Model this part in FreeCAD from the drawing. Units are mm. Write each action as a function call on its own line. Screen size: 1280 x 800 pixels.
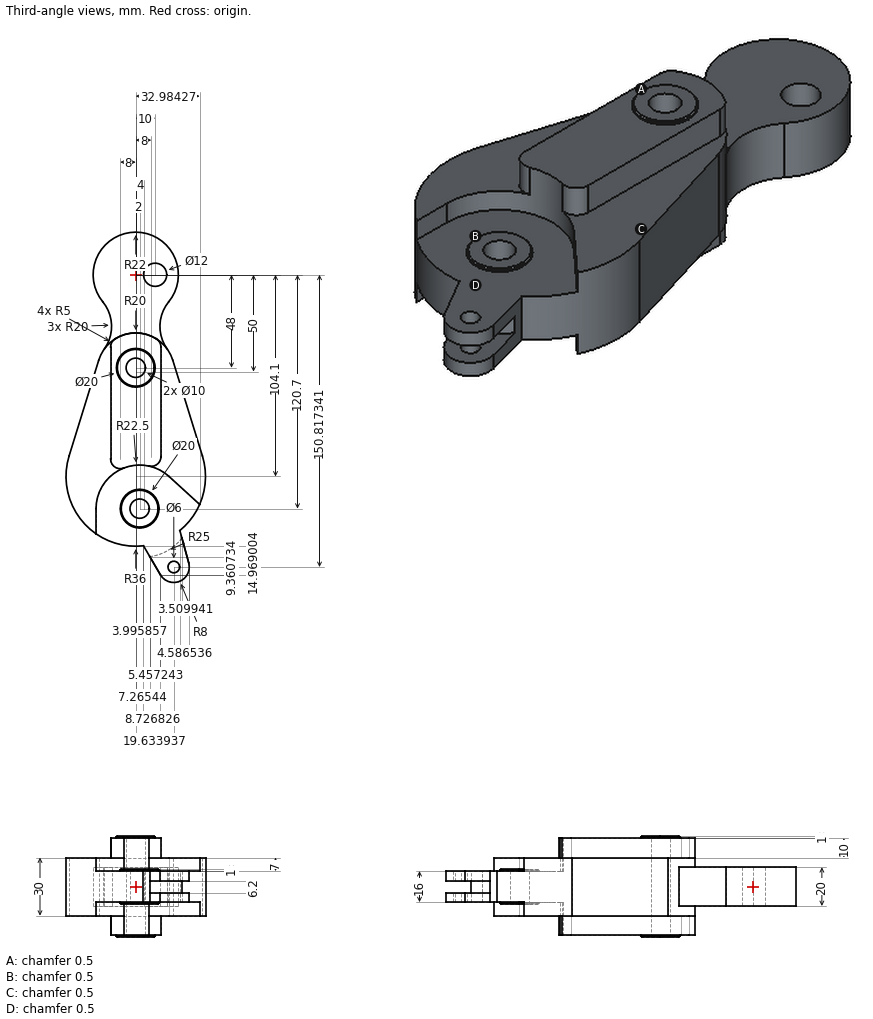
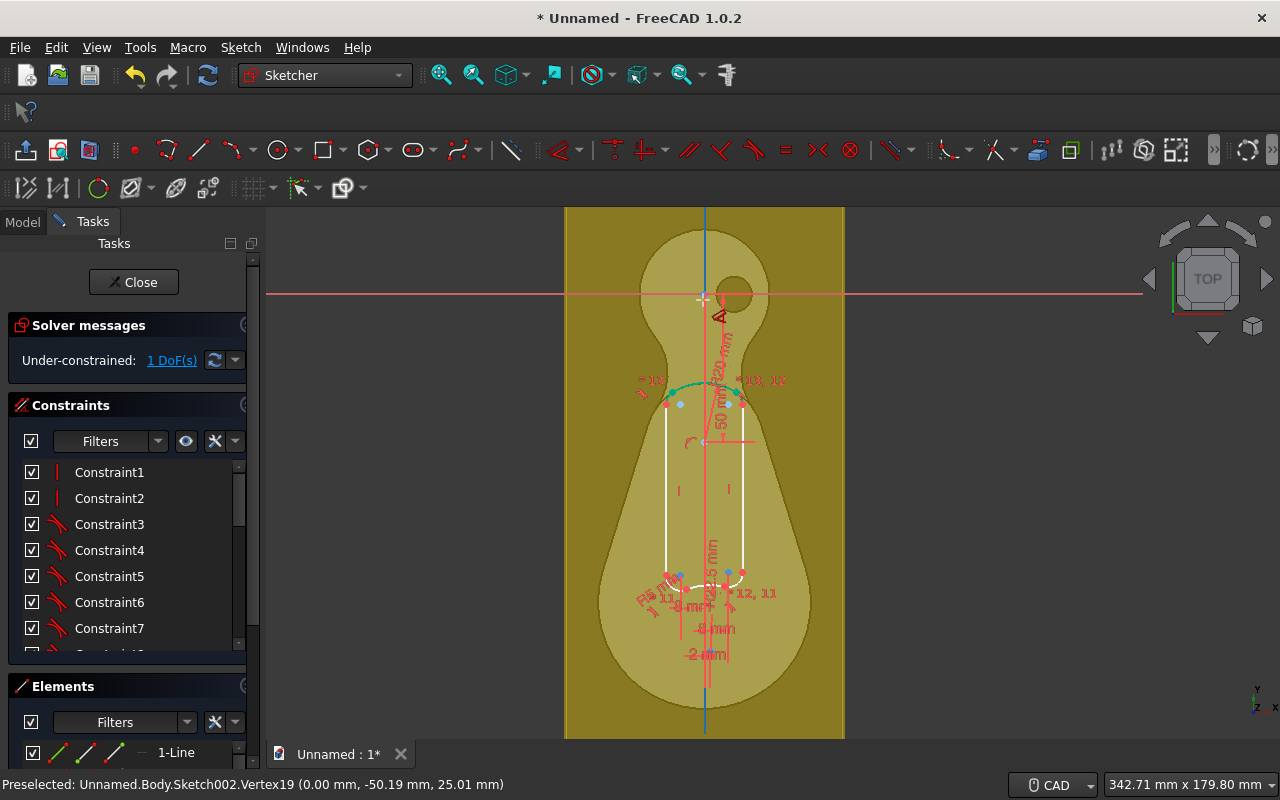
click(710, 652)
click(768, 473)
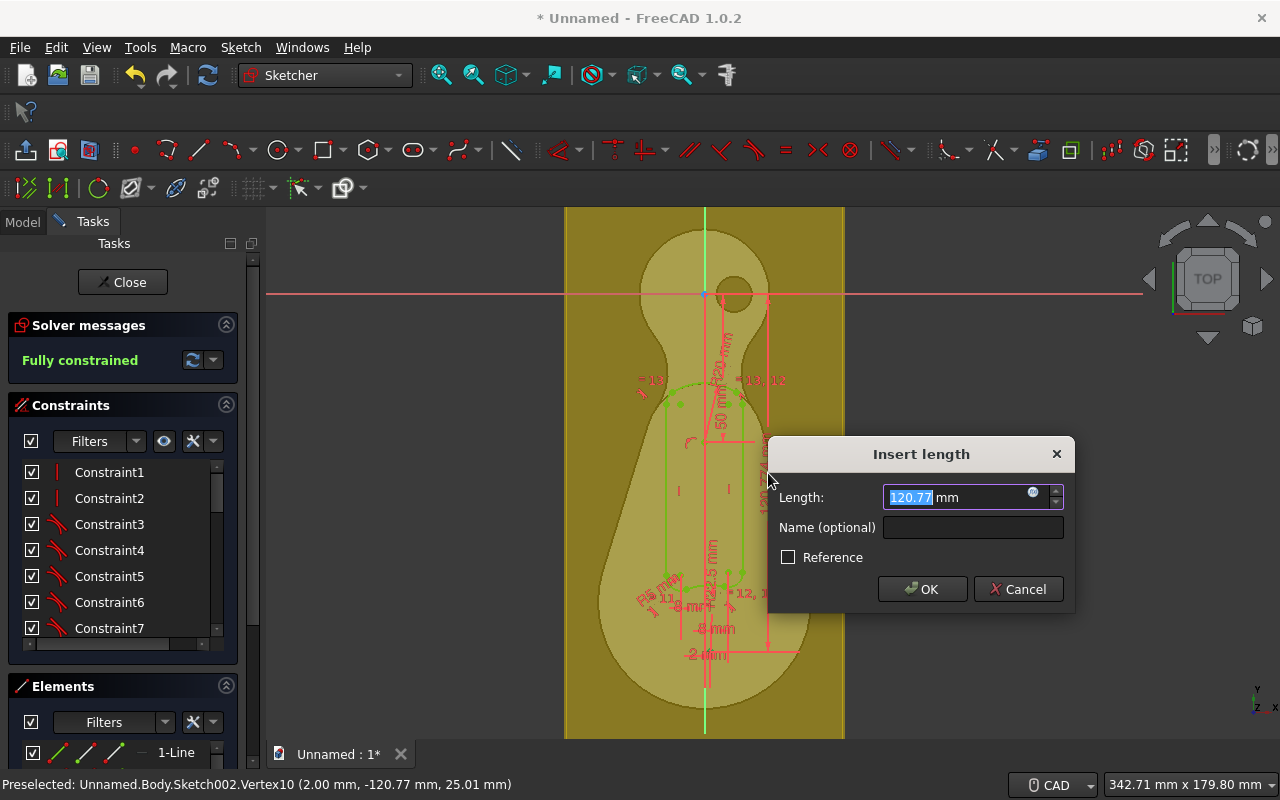
text(120.7)
key(Return)
key(Escape)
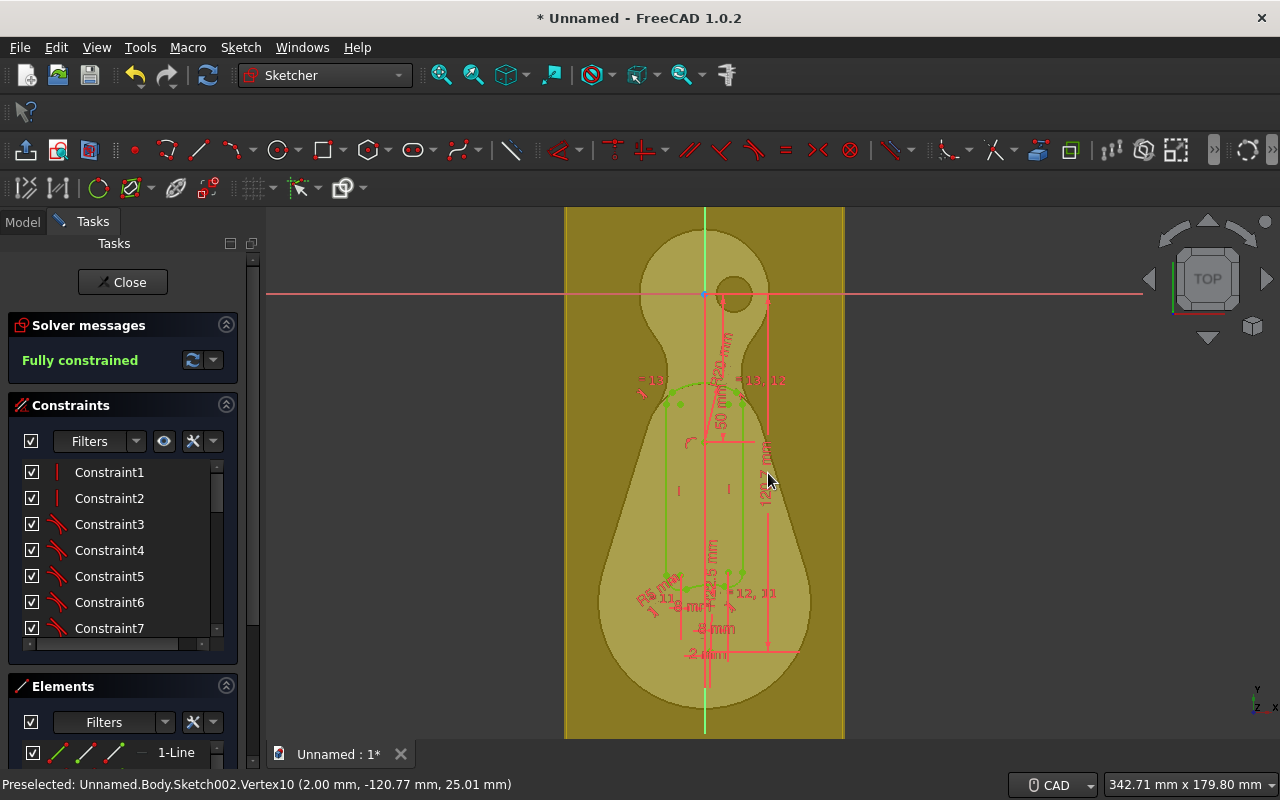
click(123, 282)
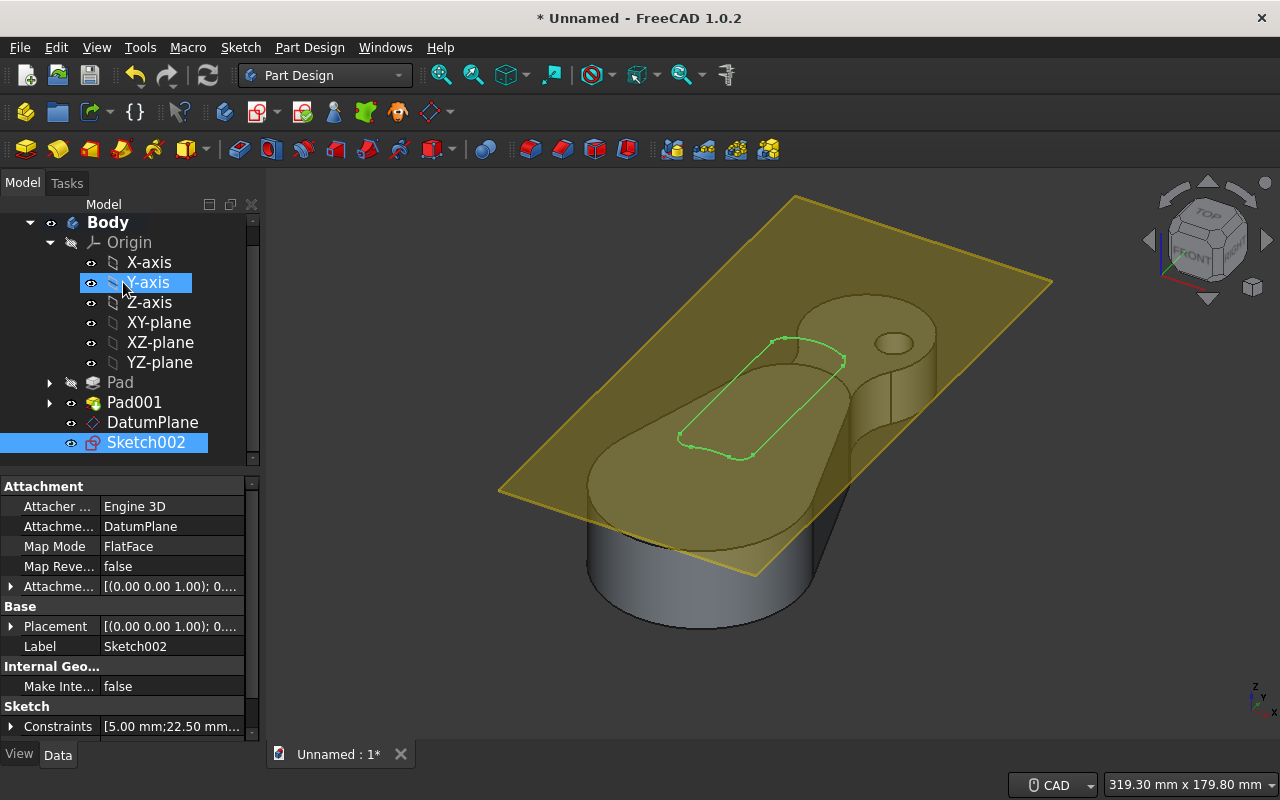
click(26, 150)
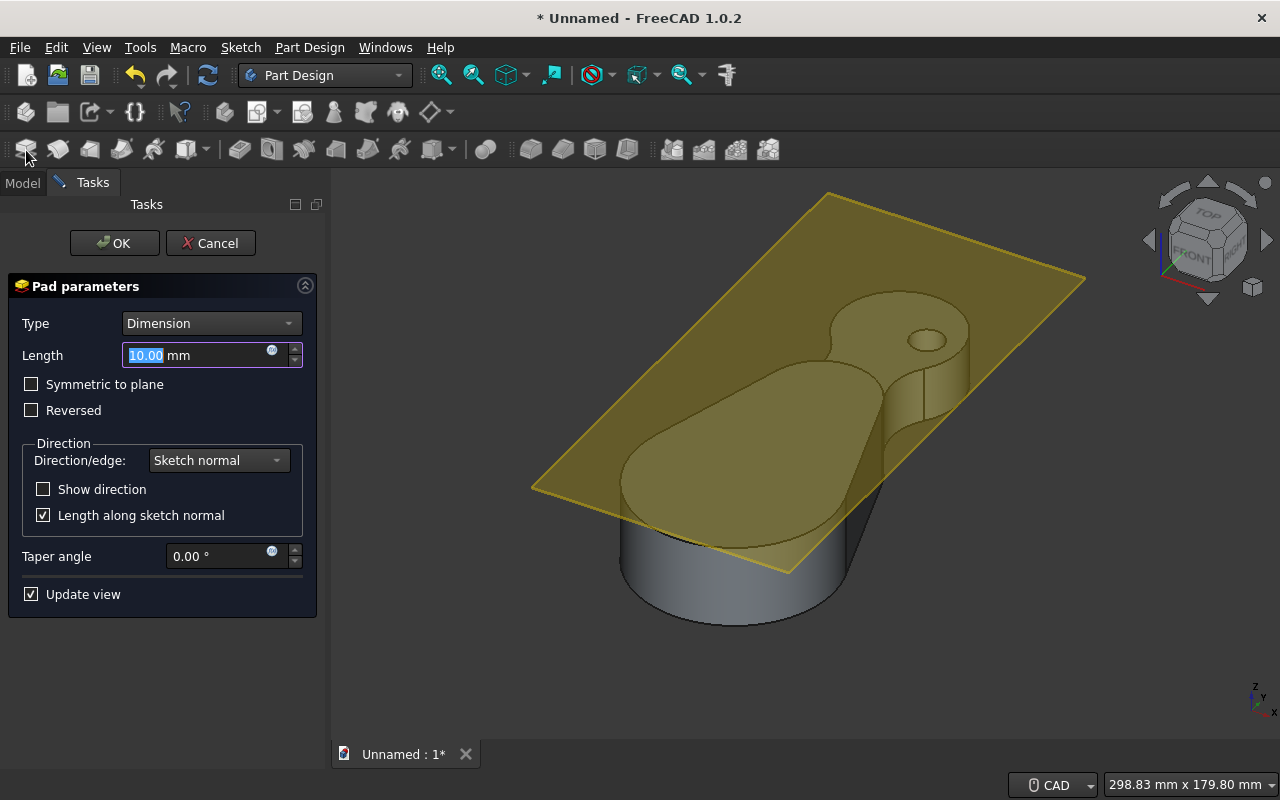
text(10)
key(Tab)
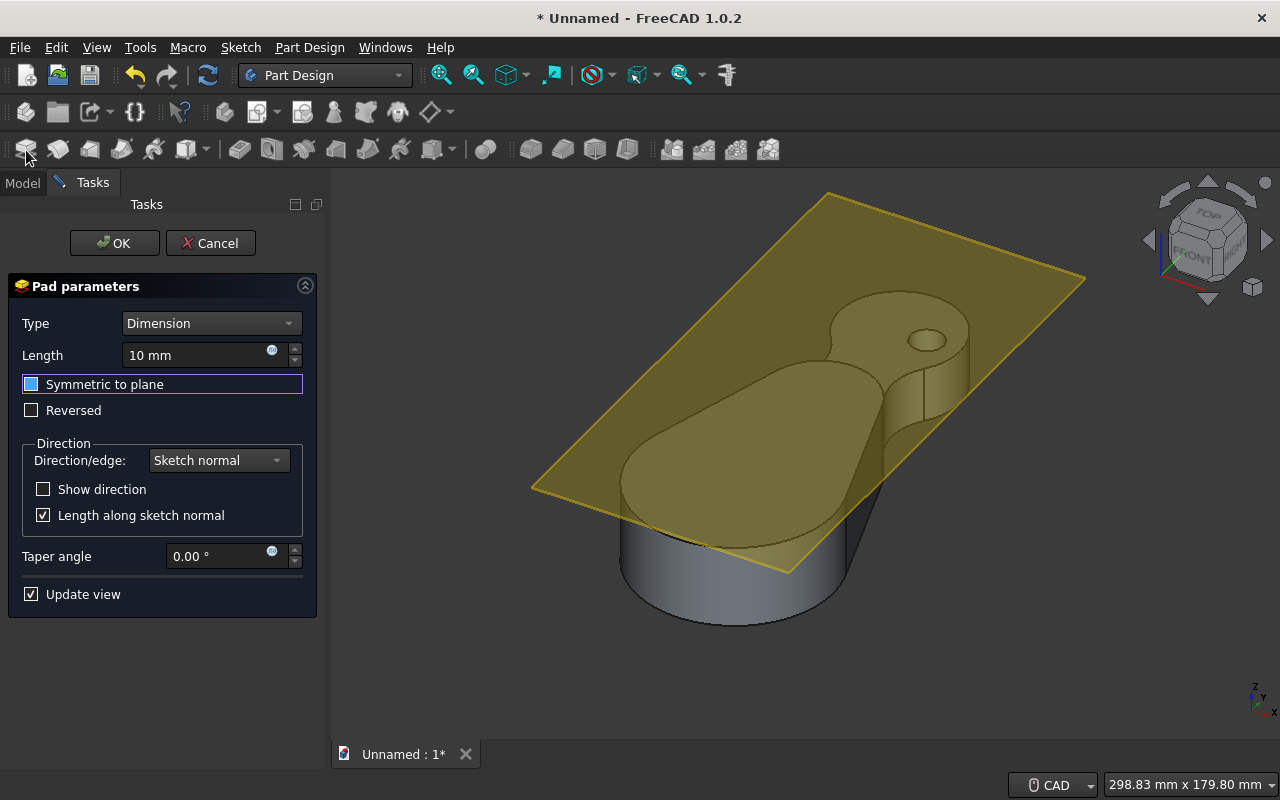
click(30, 410)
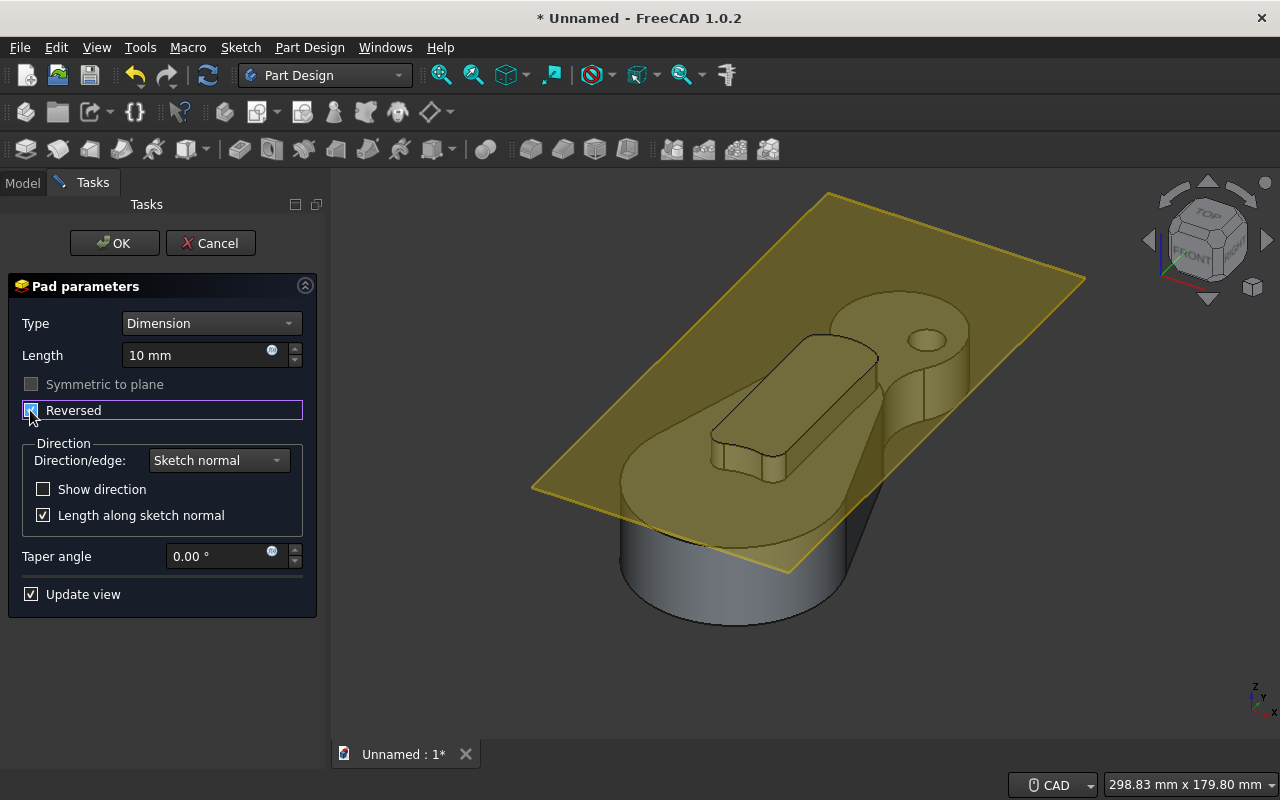
click(115, 243)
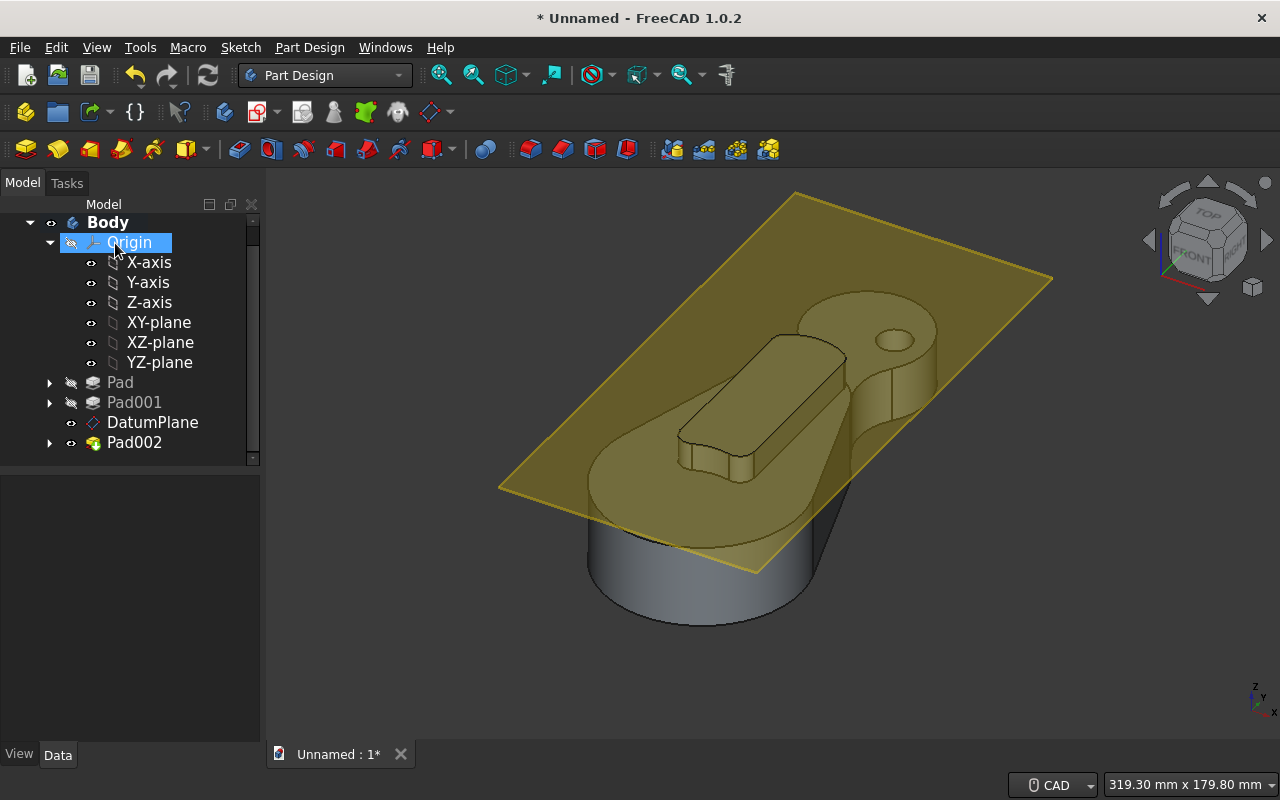
click(116, 423)
key(space)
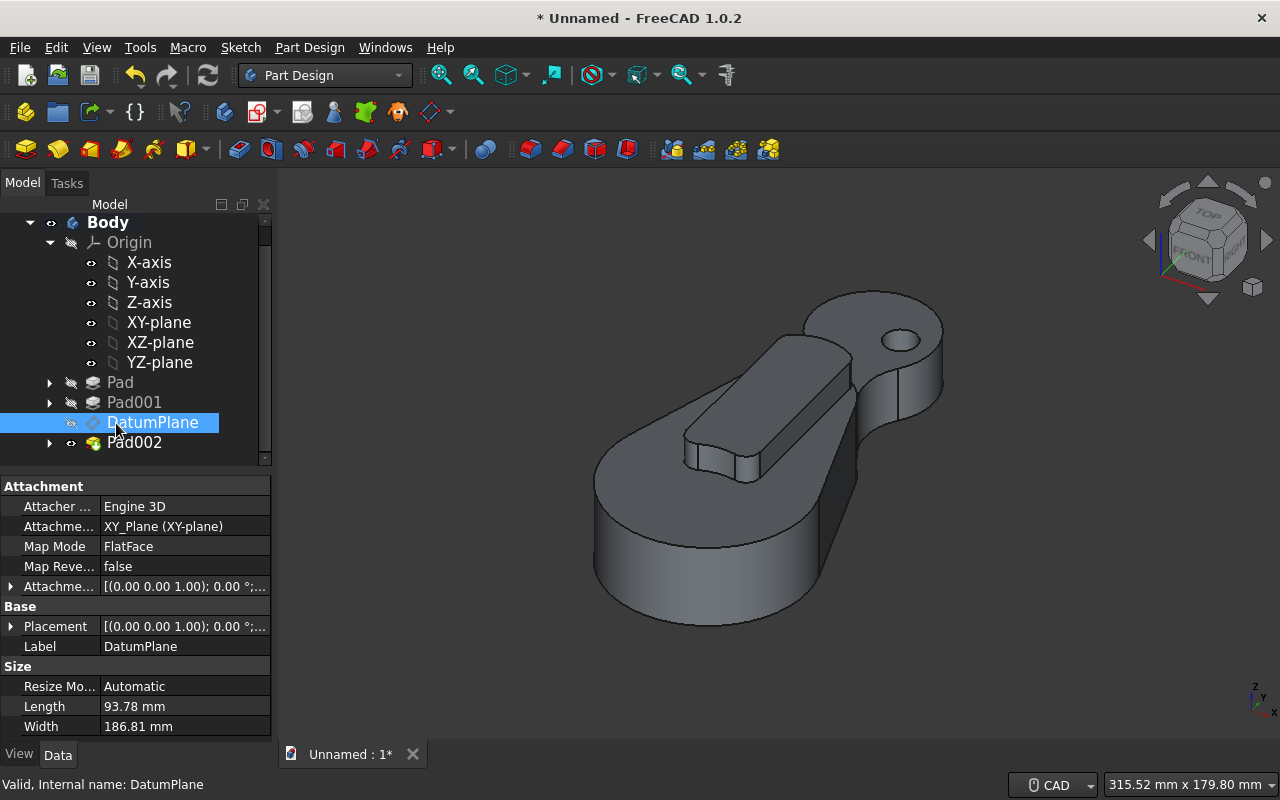
click(687, 502)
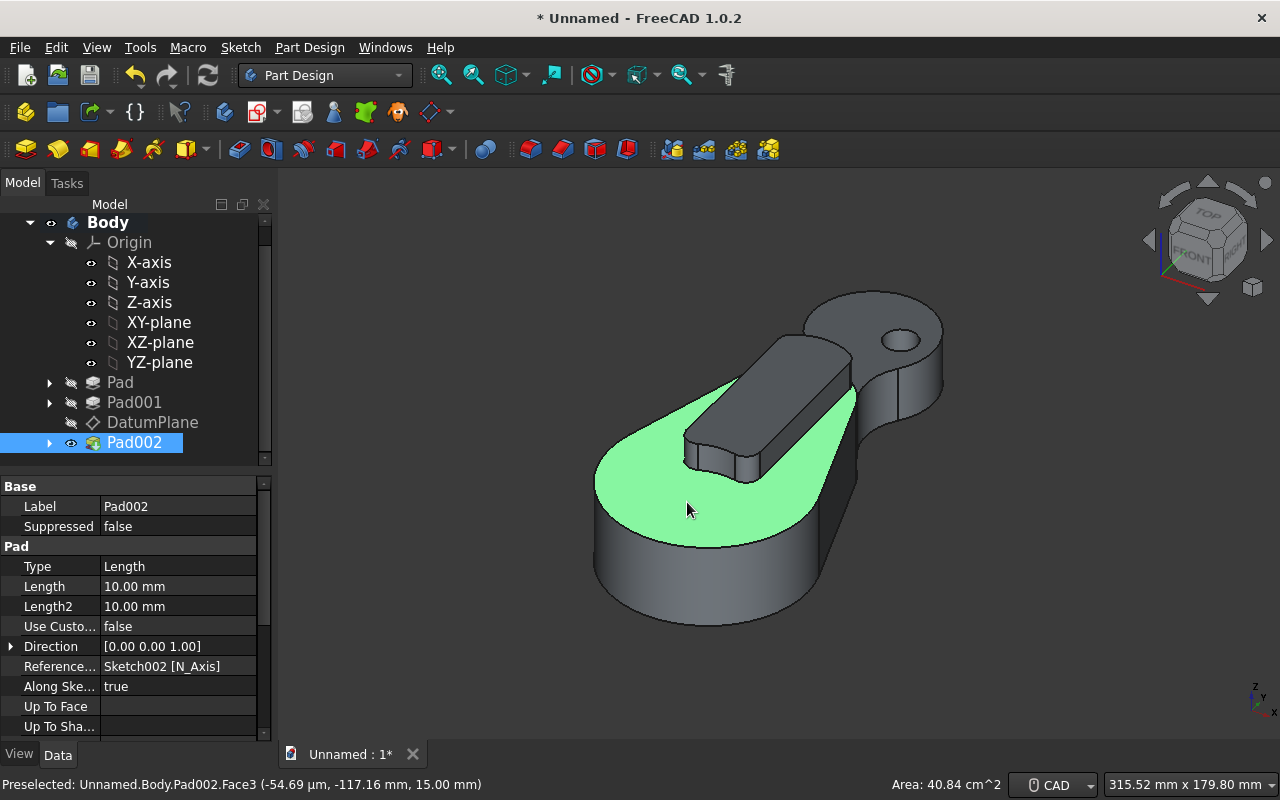
click(258, 112)